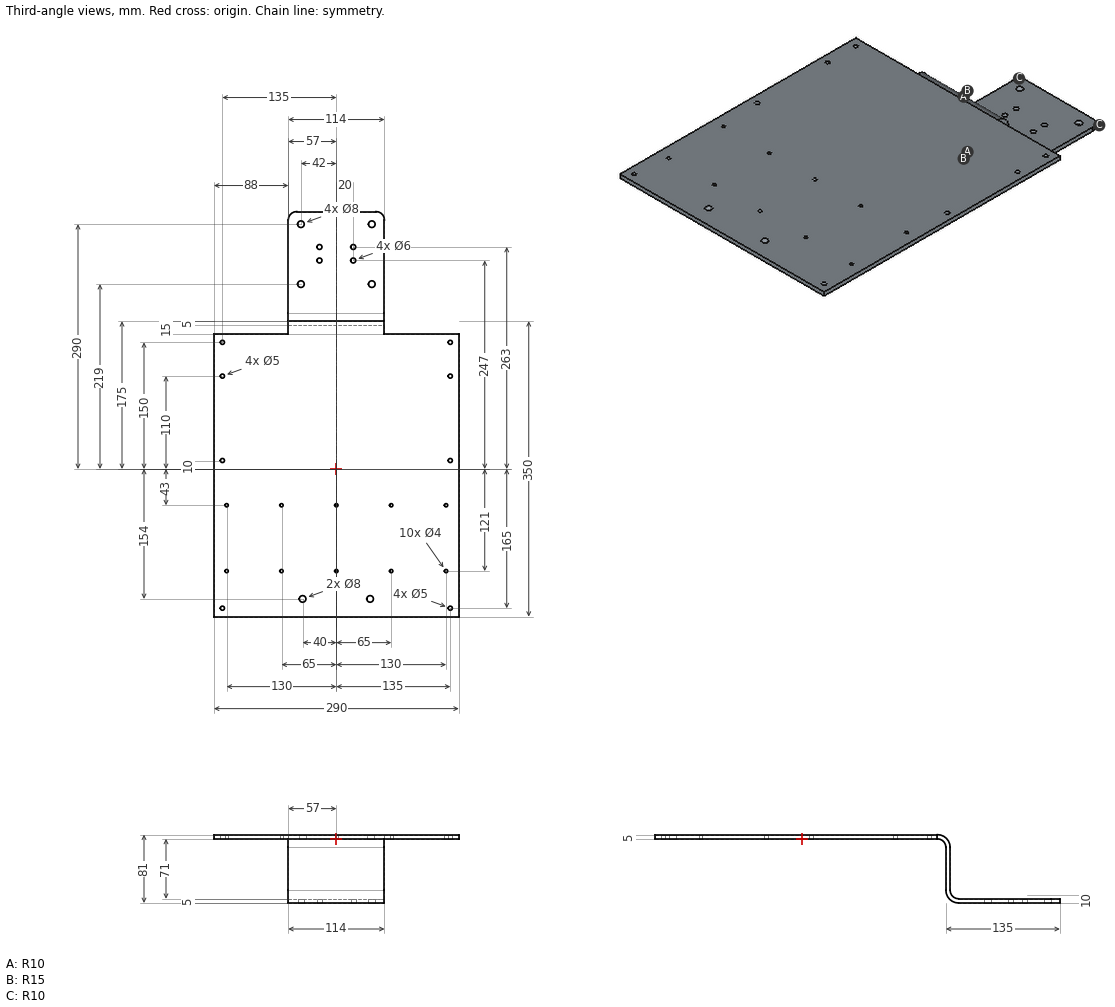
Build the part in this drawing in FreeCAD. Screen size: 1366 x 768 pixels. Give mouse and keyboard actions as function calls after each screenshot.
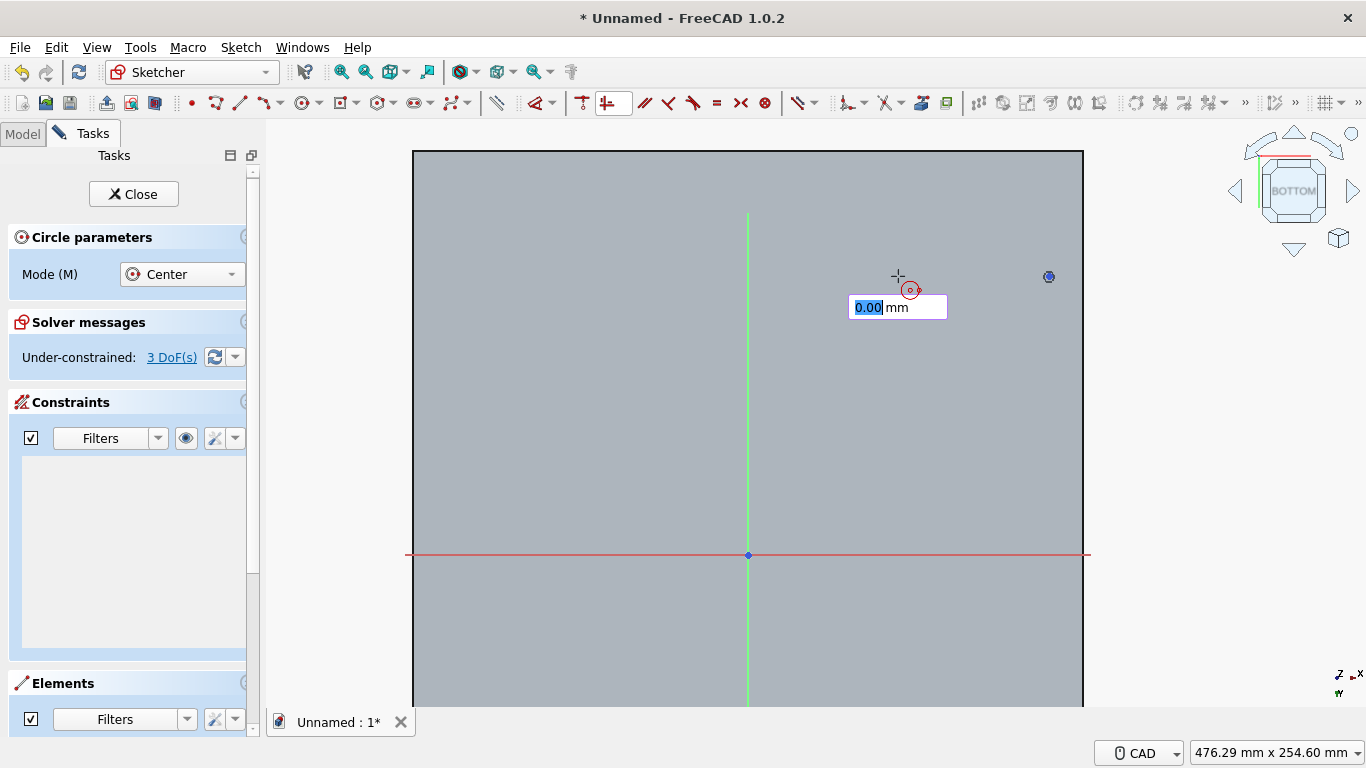
scroll(902, 273, up, 7)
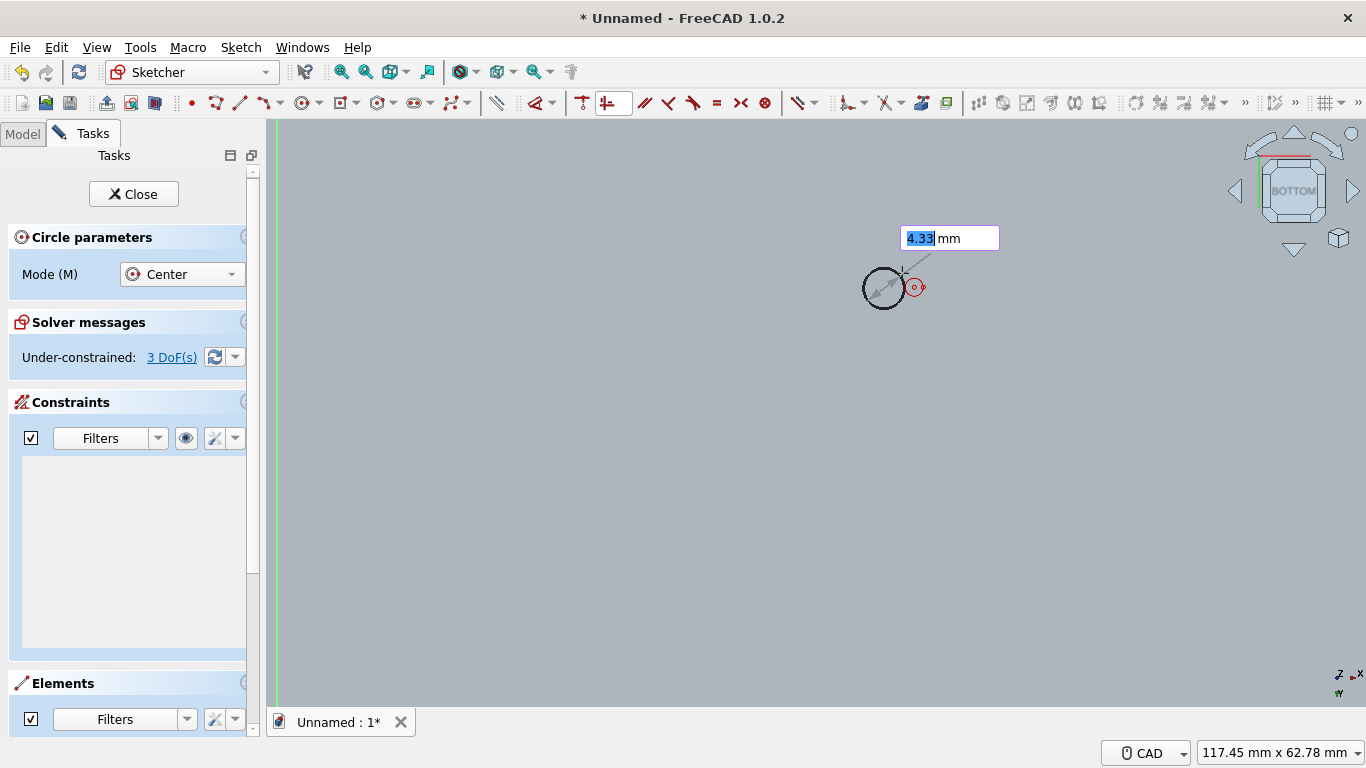
click(899, 270)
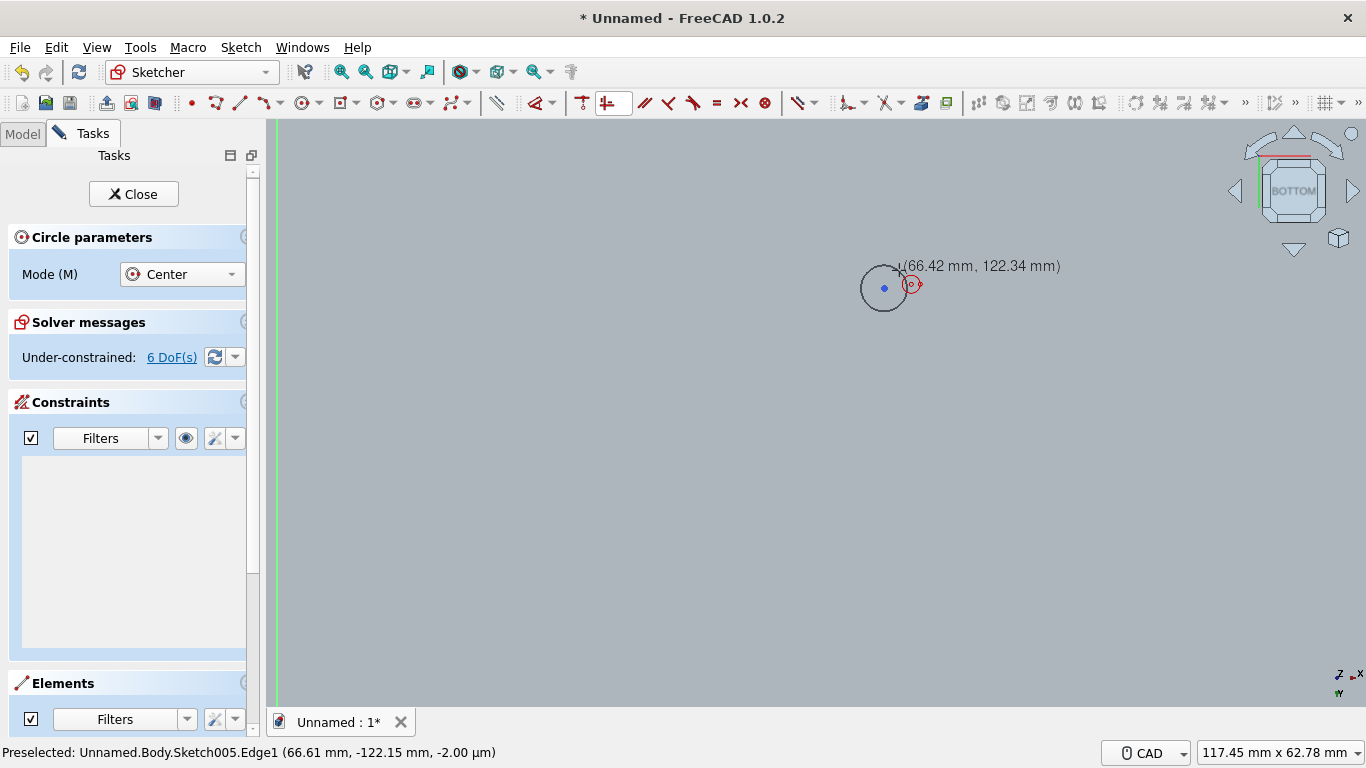
scroll(902, 273, down, 7)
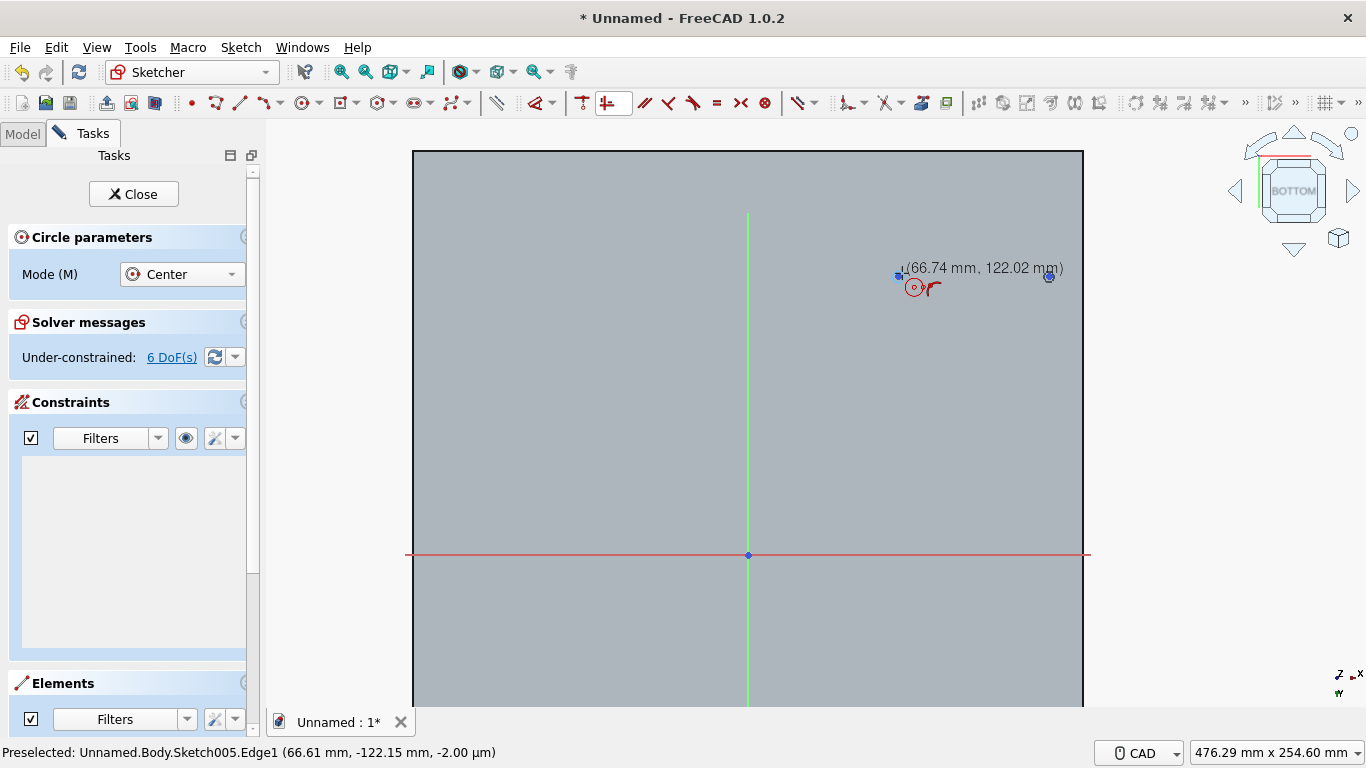
scroll(748, 276, up, 8)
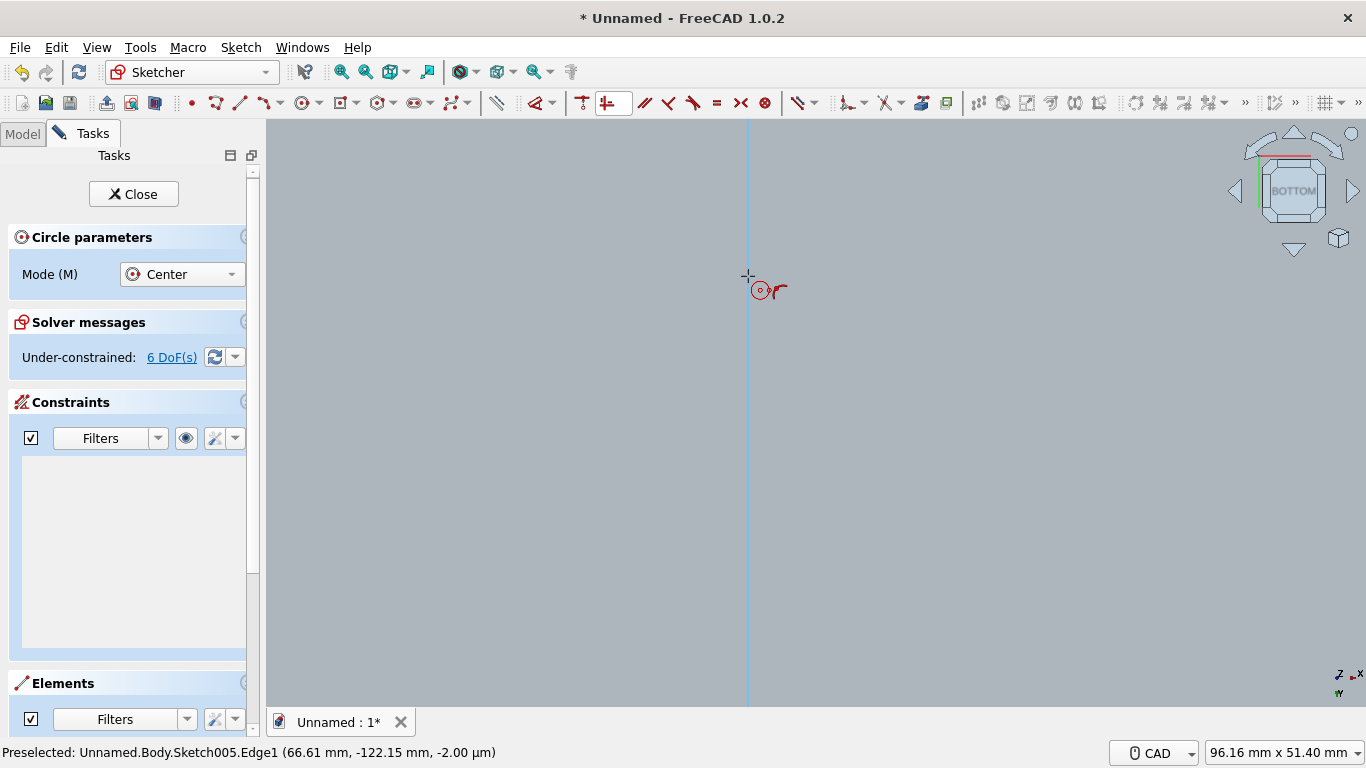
scroll(747, 276, down, 8)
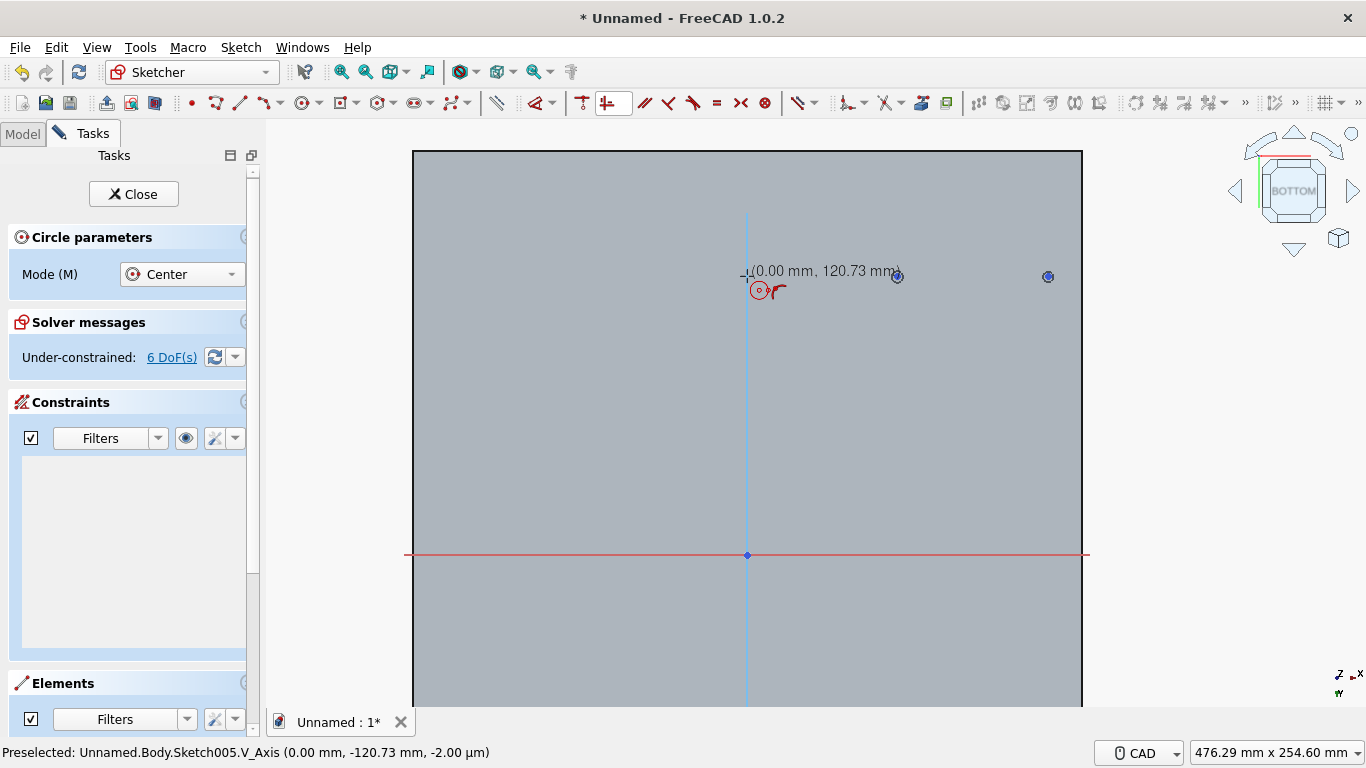
click(747, 276)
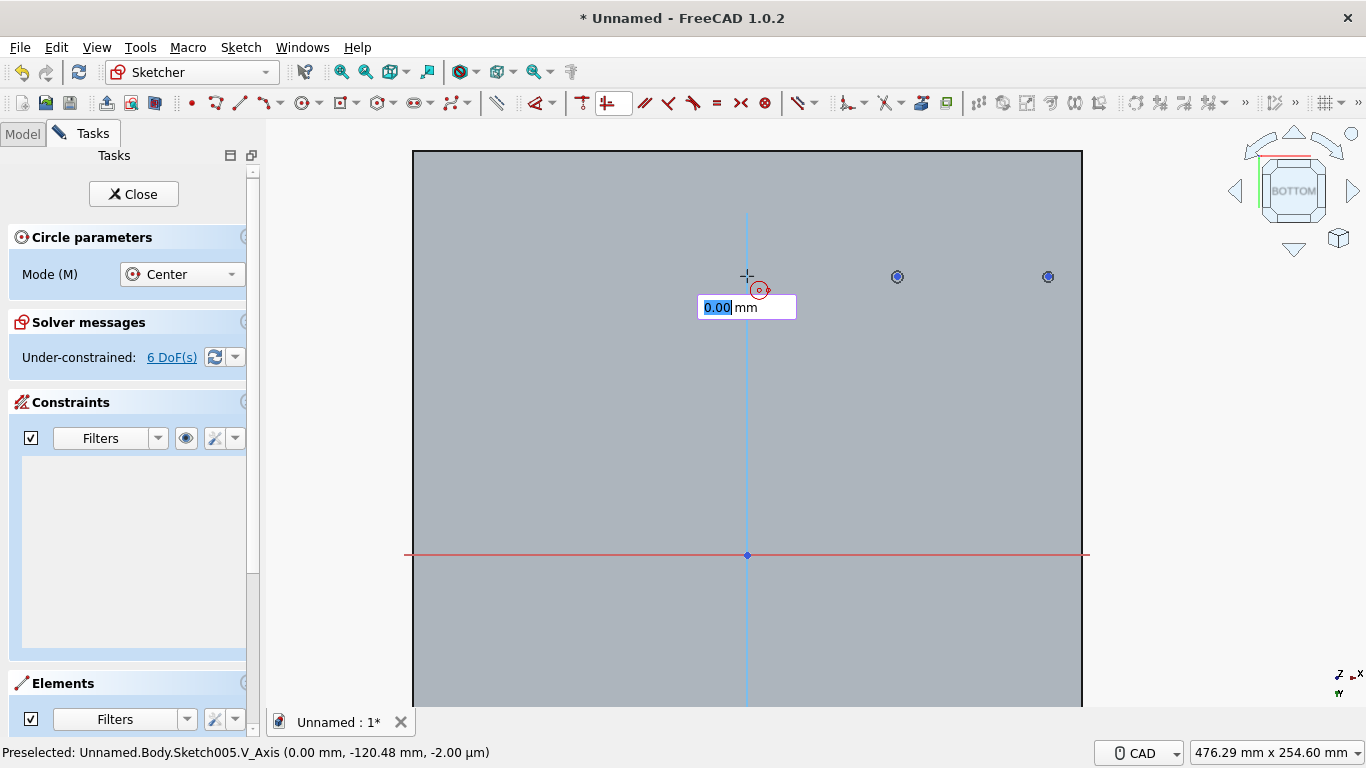
scroll(752, 274, up, 7)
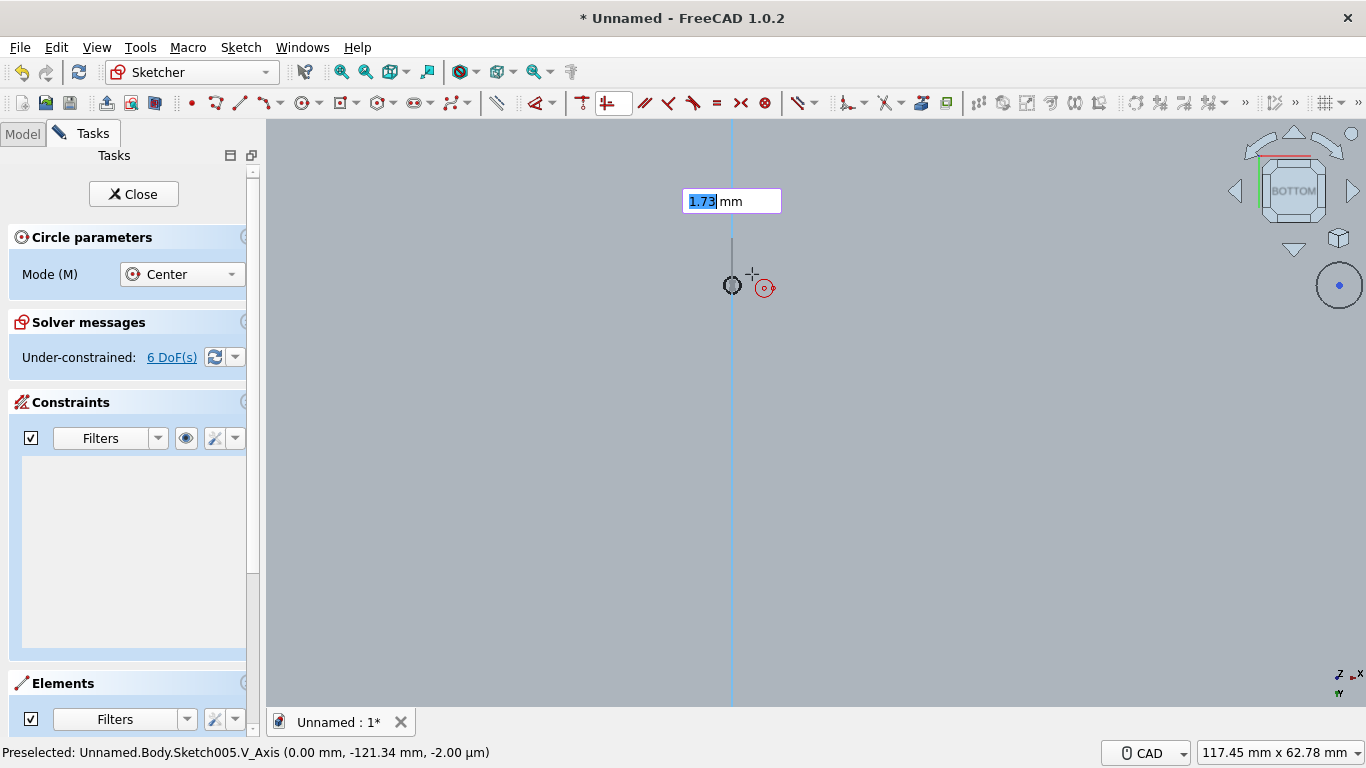
click(750, 274)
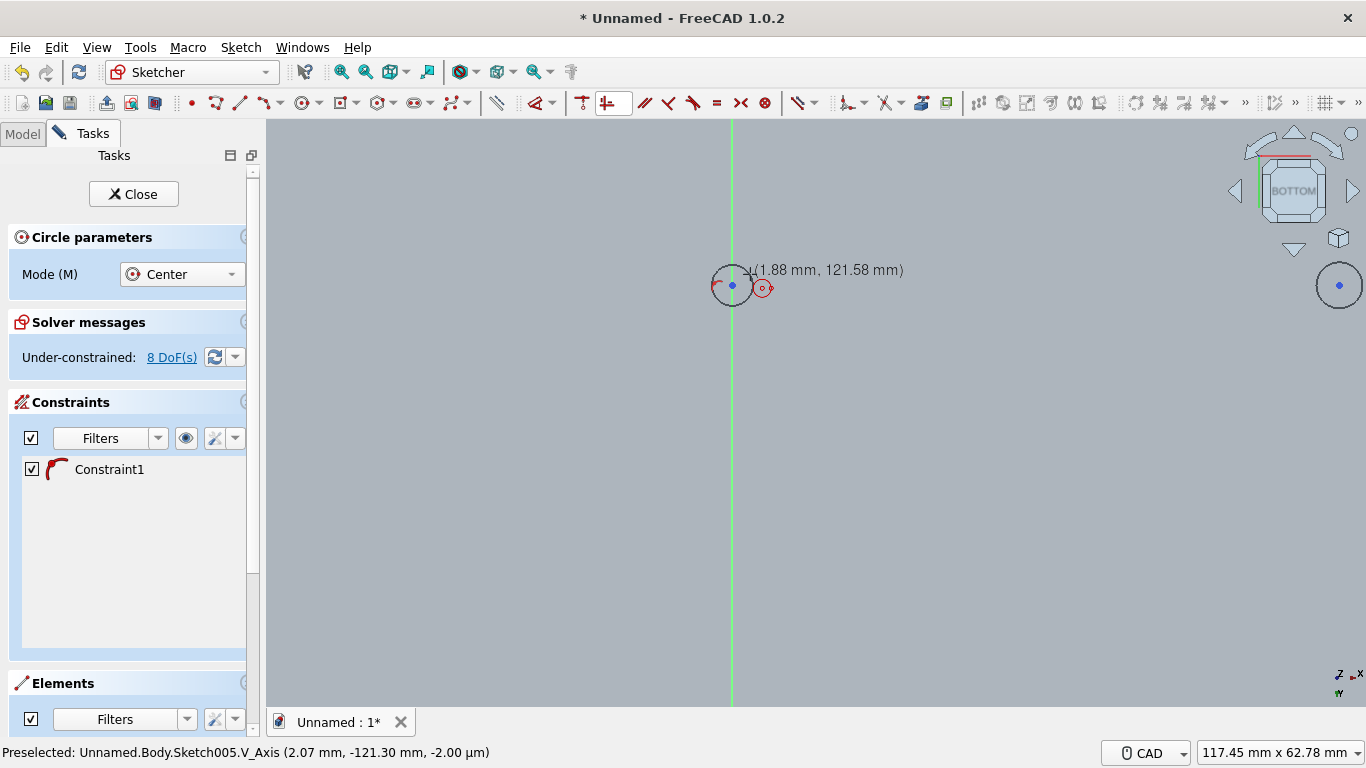
scroll(752, 274, down, 7)